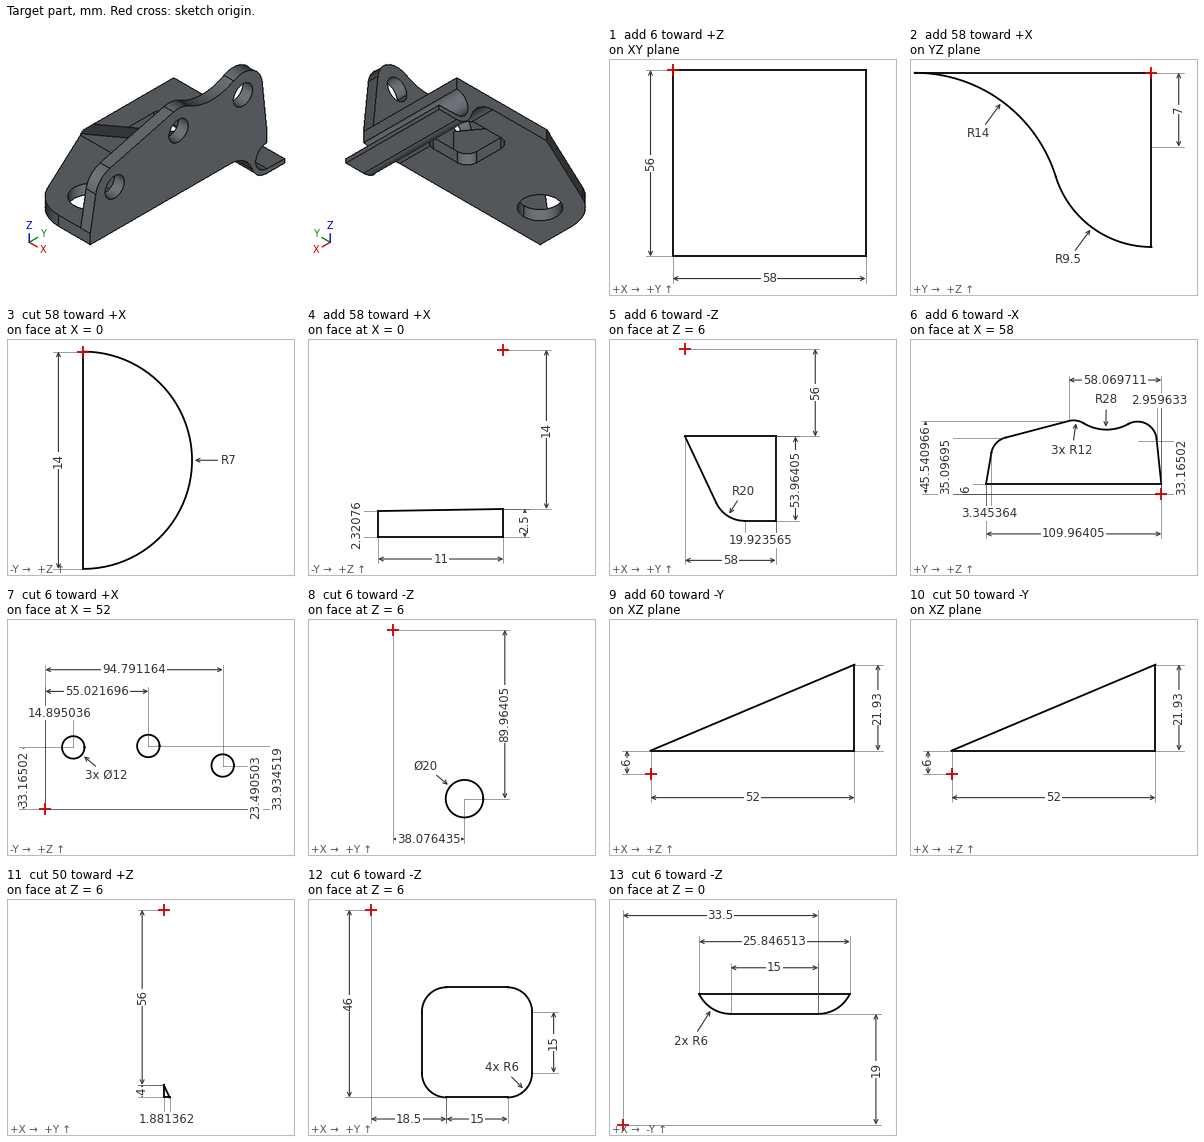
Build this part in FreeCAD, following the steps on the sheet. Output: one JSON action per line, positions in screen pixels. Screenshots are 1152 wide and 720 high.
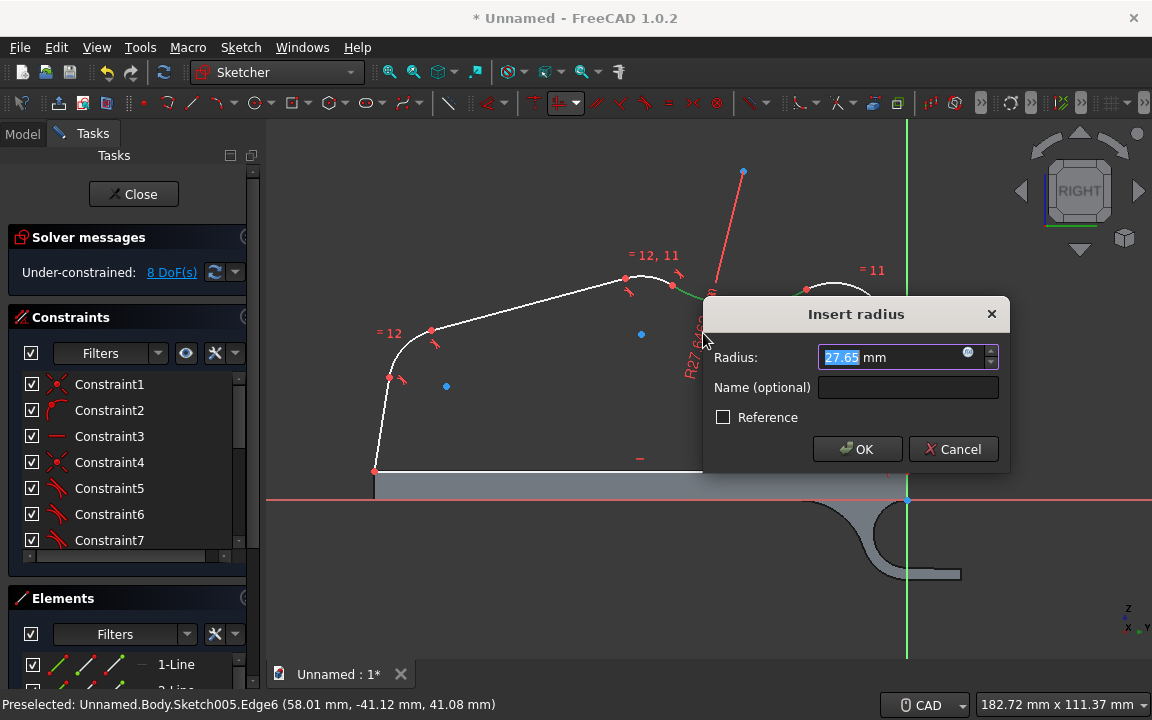
{"action": "type", "text": "28"}
{"action": "key", "text": "Return"}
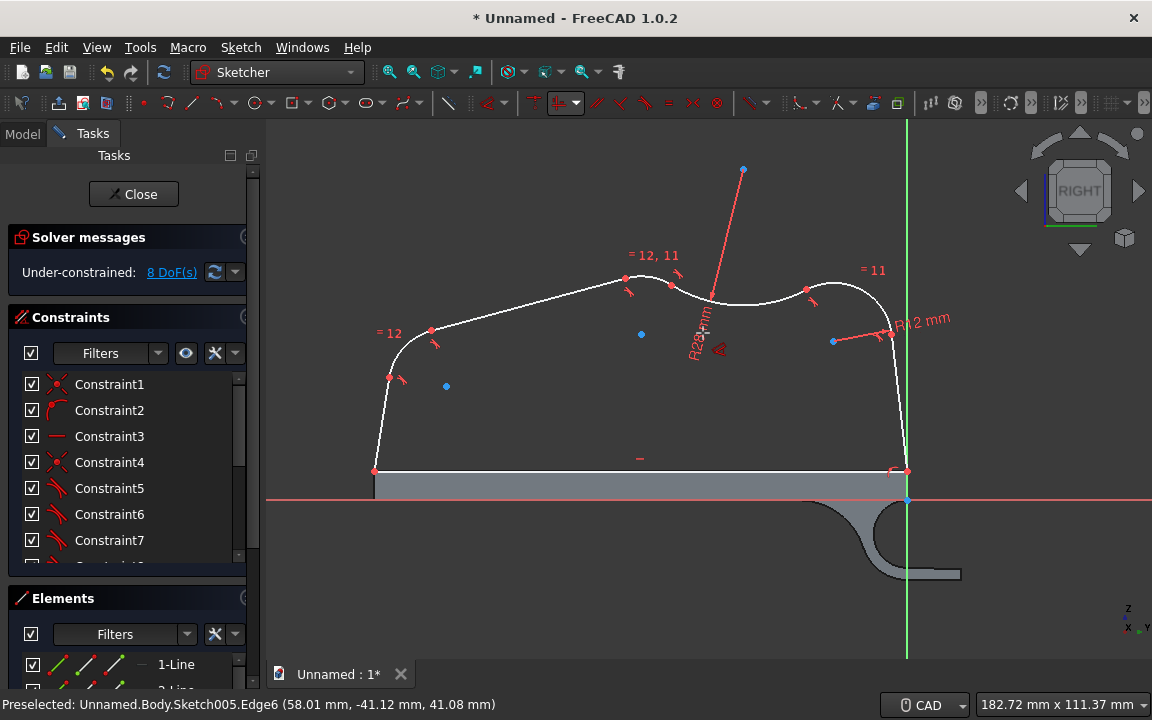
{"action": "scroll", "coordinate": [374, 472], "scroll_direction": "up", "scroll_amount": 2}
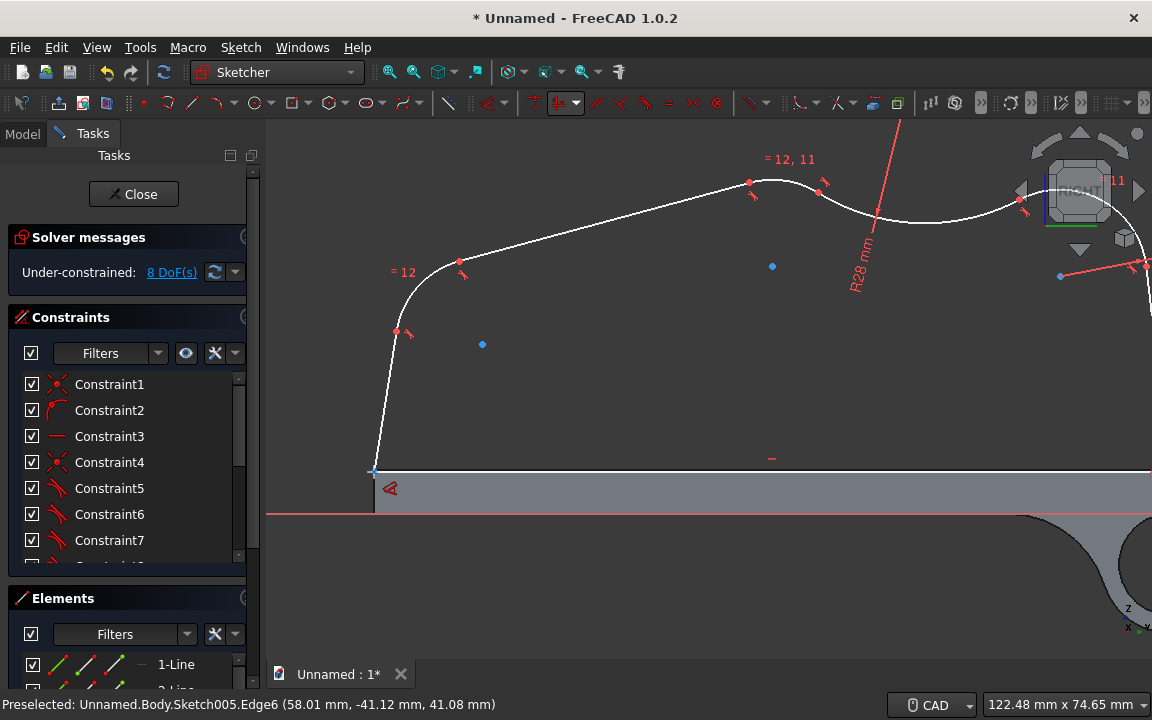
{"action": "left_click", "coordinate": [374, 472]}
{"action": "left_click", "coordinate": [340, 493]}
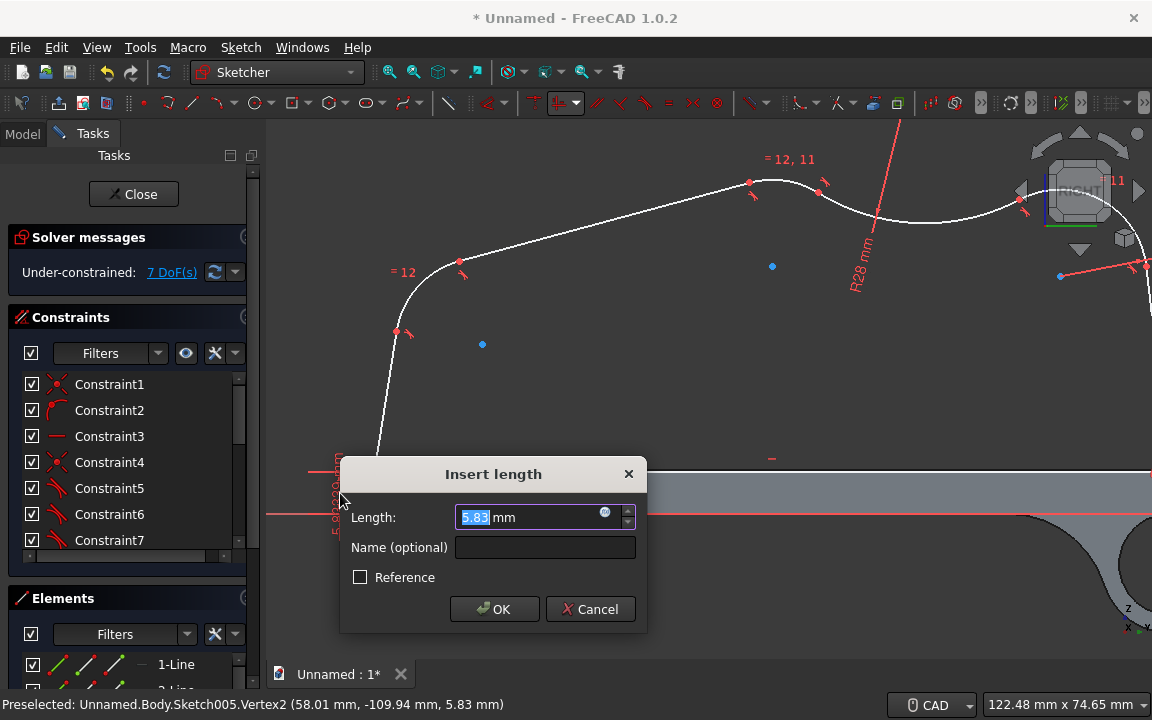
{"action": "type", "text": "6"}
{"action": "key", "text": "Return"}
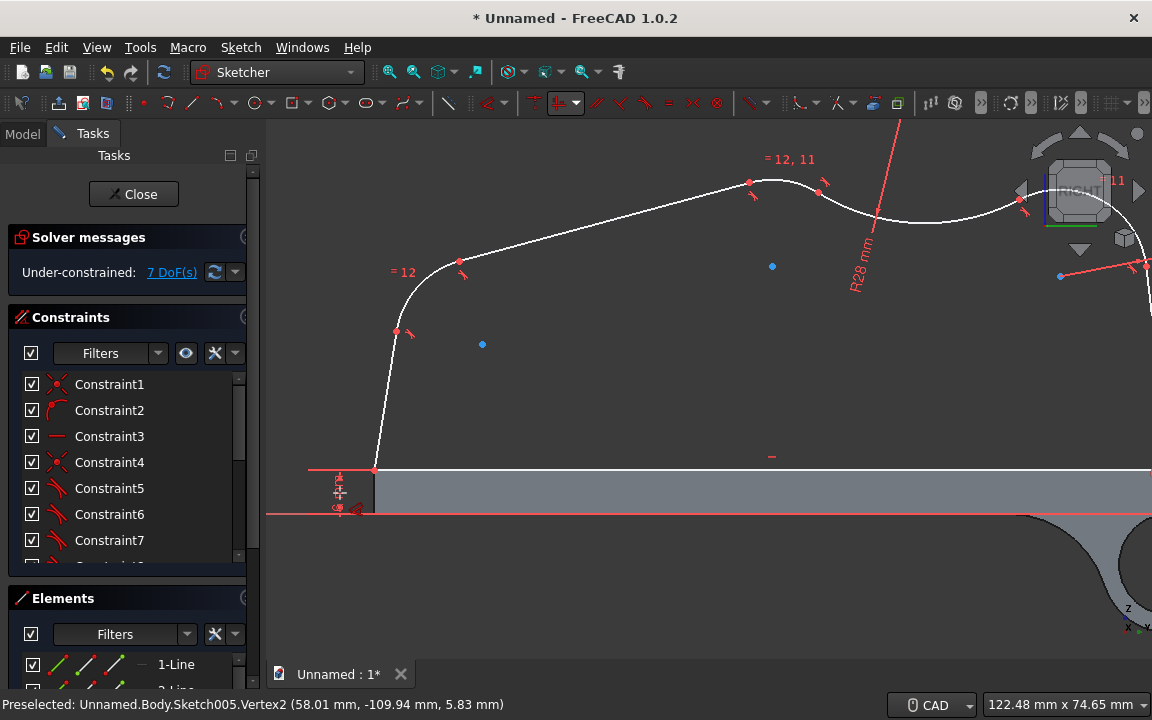
{"action": "left_click", "coordinate": [613, 470]}
{"action": "left_click", "coordinate": [681, 436]}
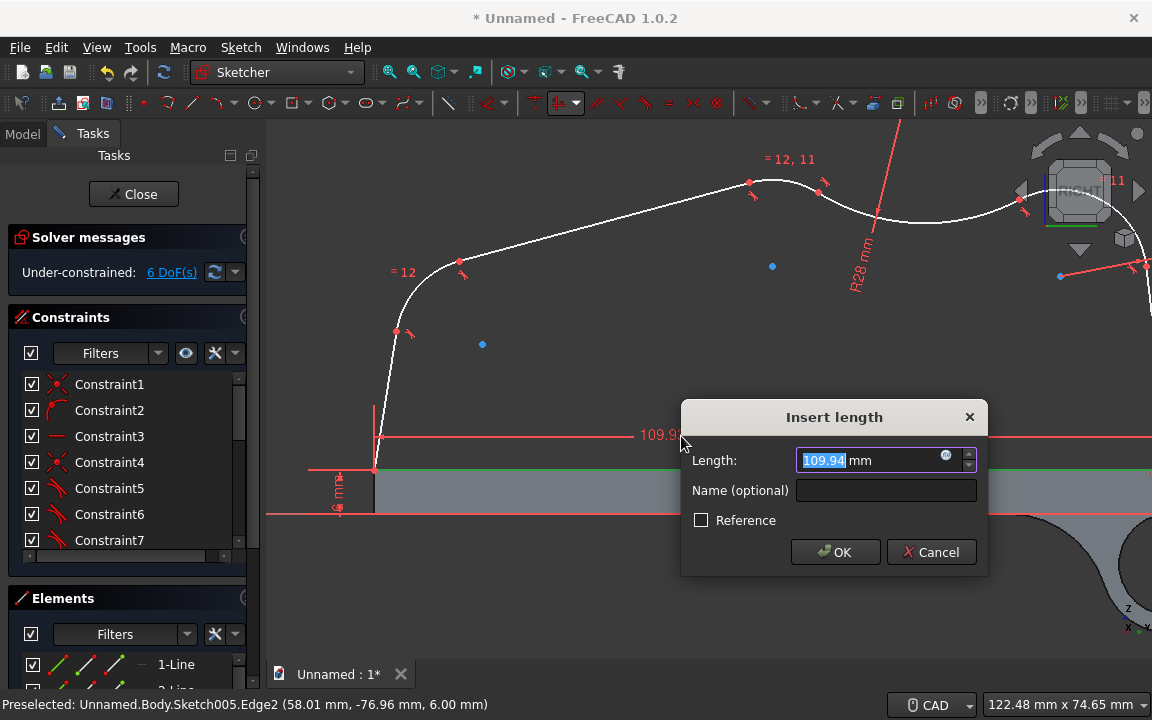
{"action": "type", "text": "109.96405"}
{"action": "key", "text": "Return"}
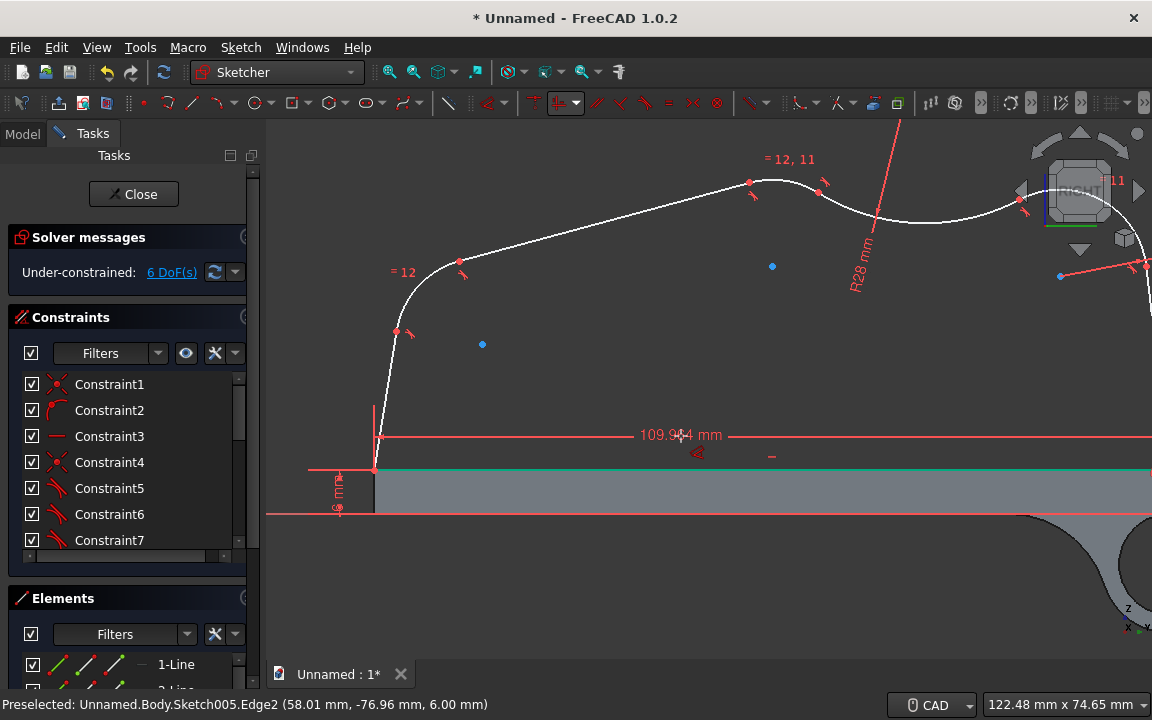
{"action": "scroll", "coordinate": [373, 472], "scroll_direction": "down", "scroll_amount": 2}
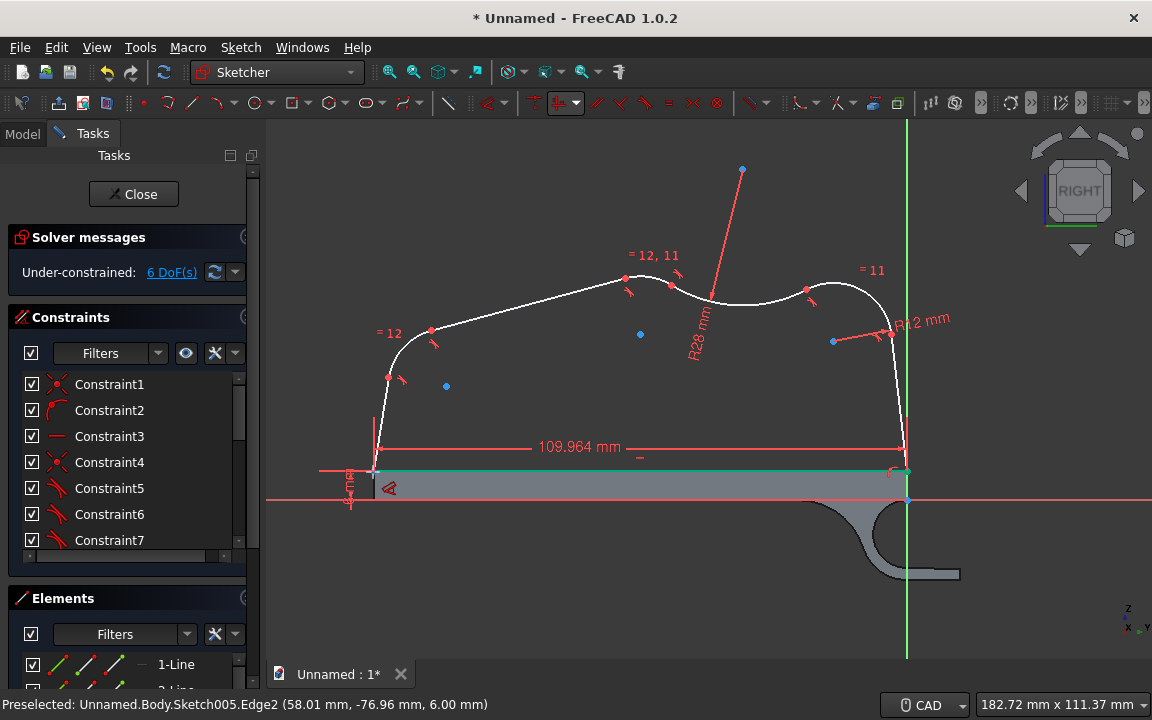
{"action": "scroll", "coordinate": [891, 335], "scroll_direction": "up", "scroll_amount": 6}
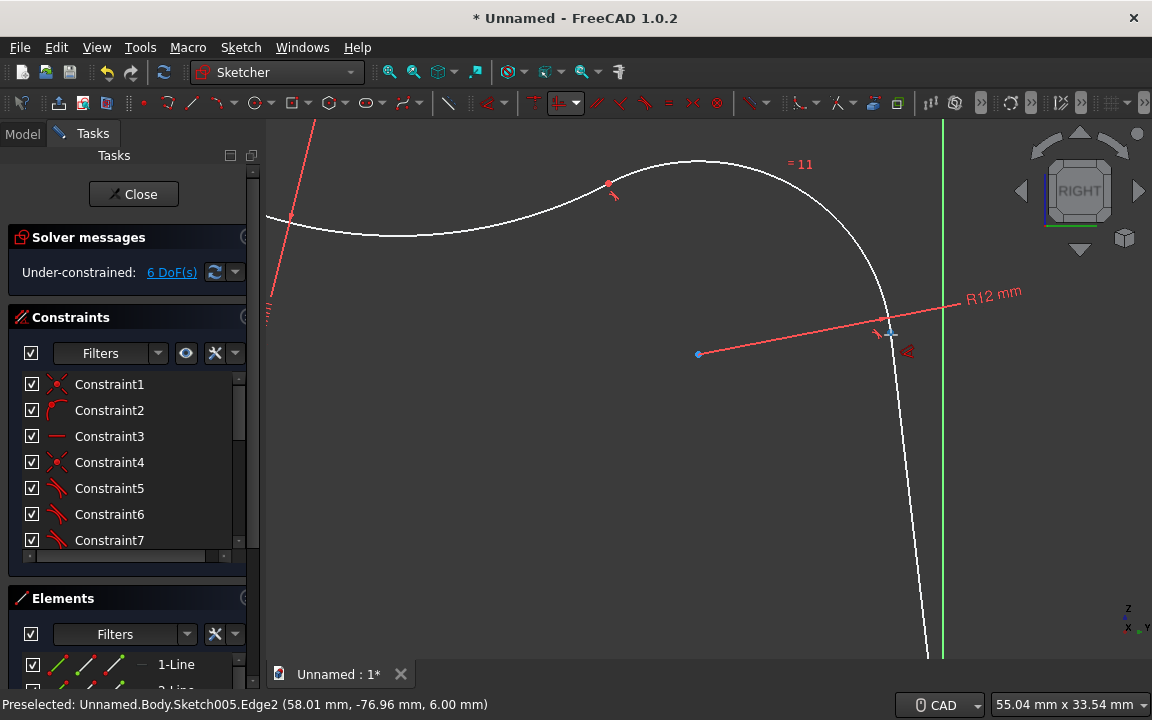
{"action": "left_click", "coordinate": [891, 332]}
{"action": "left_click", "coordinate": [917, 298]}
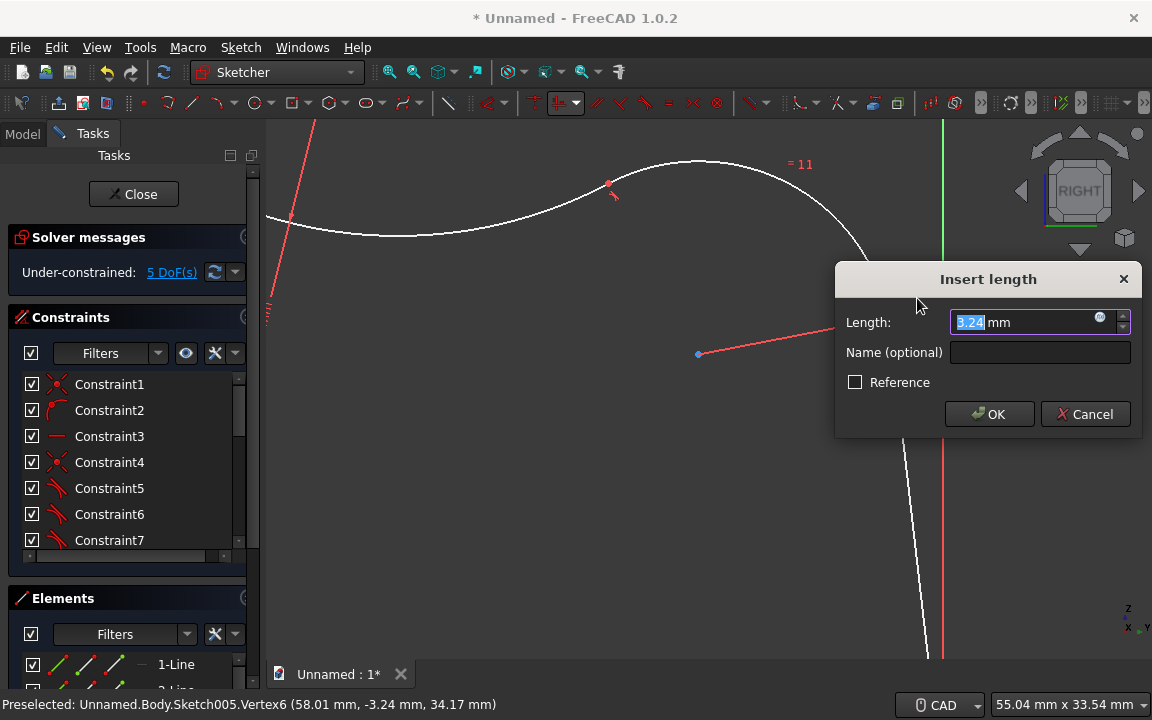
{"action": "type", "text": "2.959633"}
{"action": "key", "text": "Return"}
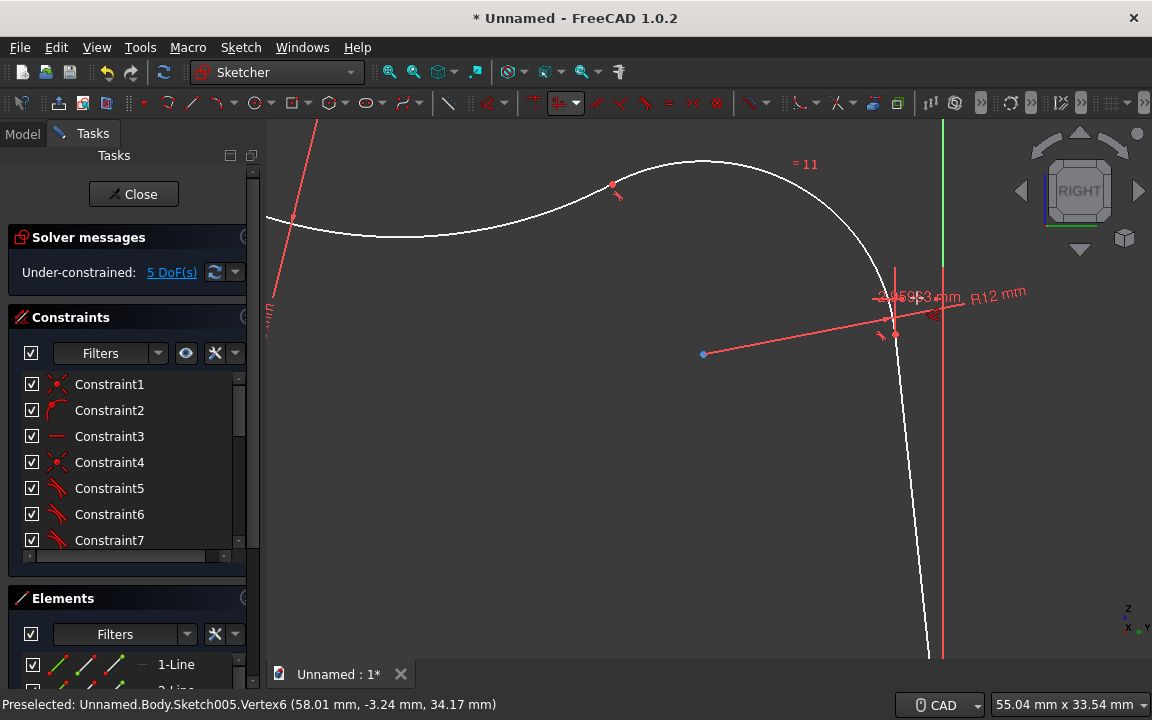
{"action": "scroll", "coordinate": [892, 335], "scroll_direction": "down", "scroll_amount": 6}